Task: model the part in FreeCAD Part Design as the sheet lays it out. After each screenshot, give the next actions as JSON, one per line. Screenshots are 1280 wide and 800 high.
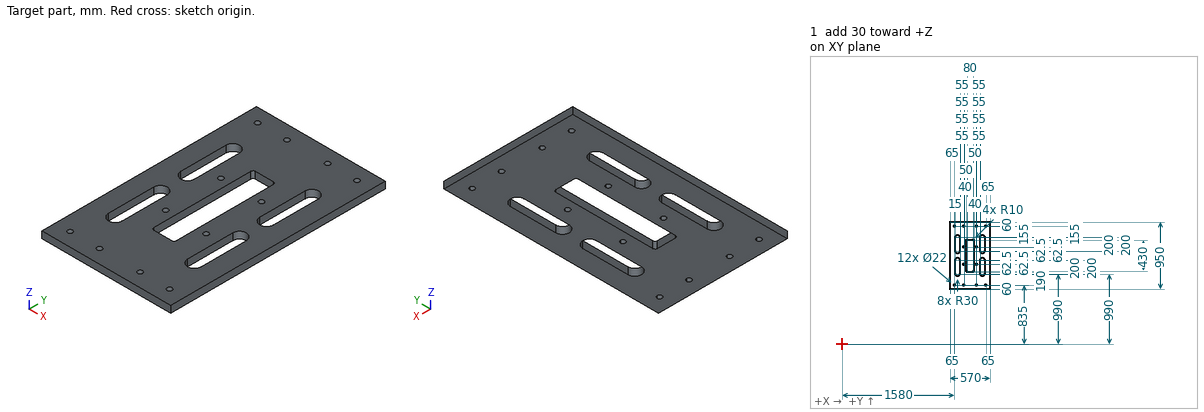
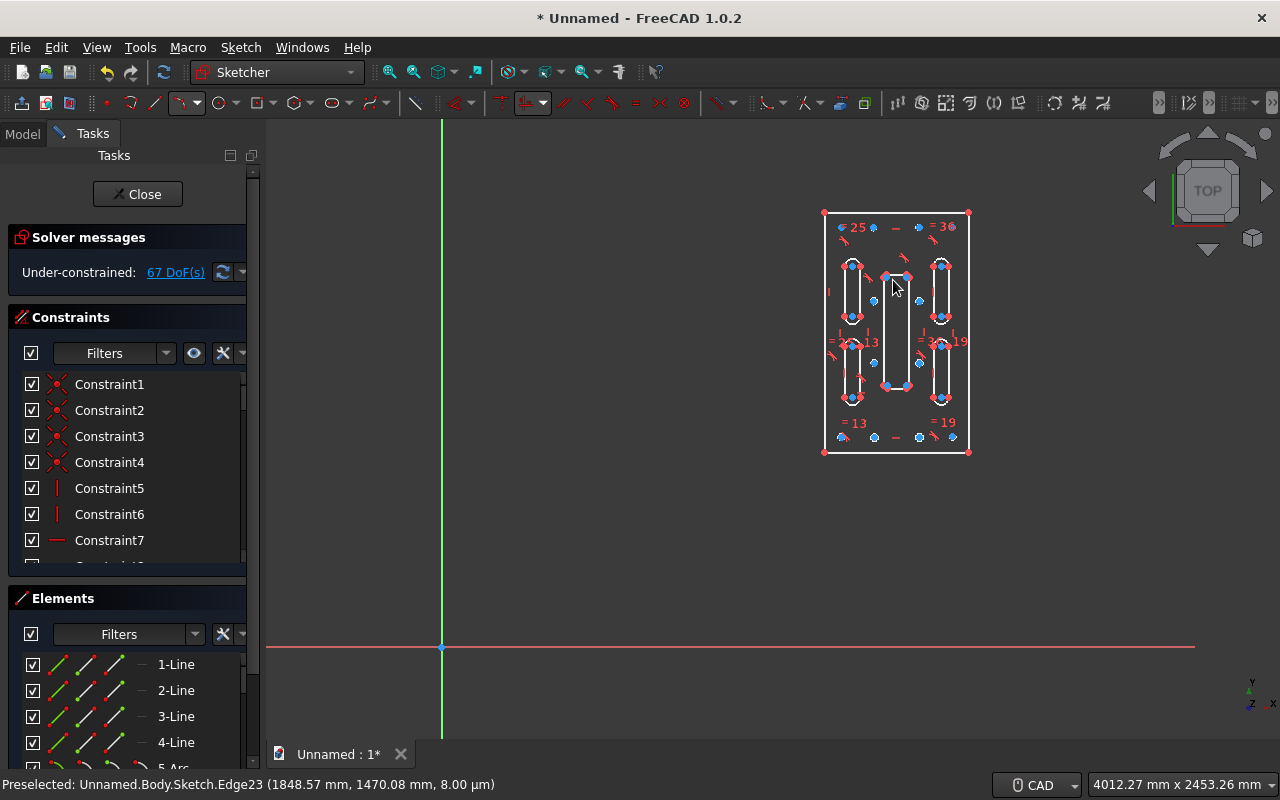
{"action": "scroll", "coordinate": [909, 310], "scroll_direction": "up", "scroll_amount": 2}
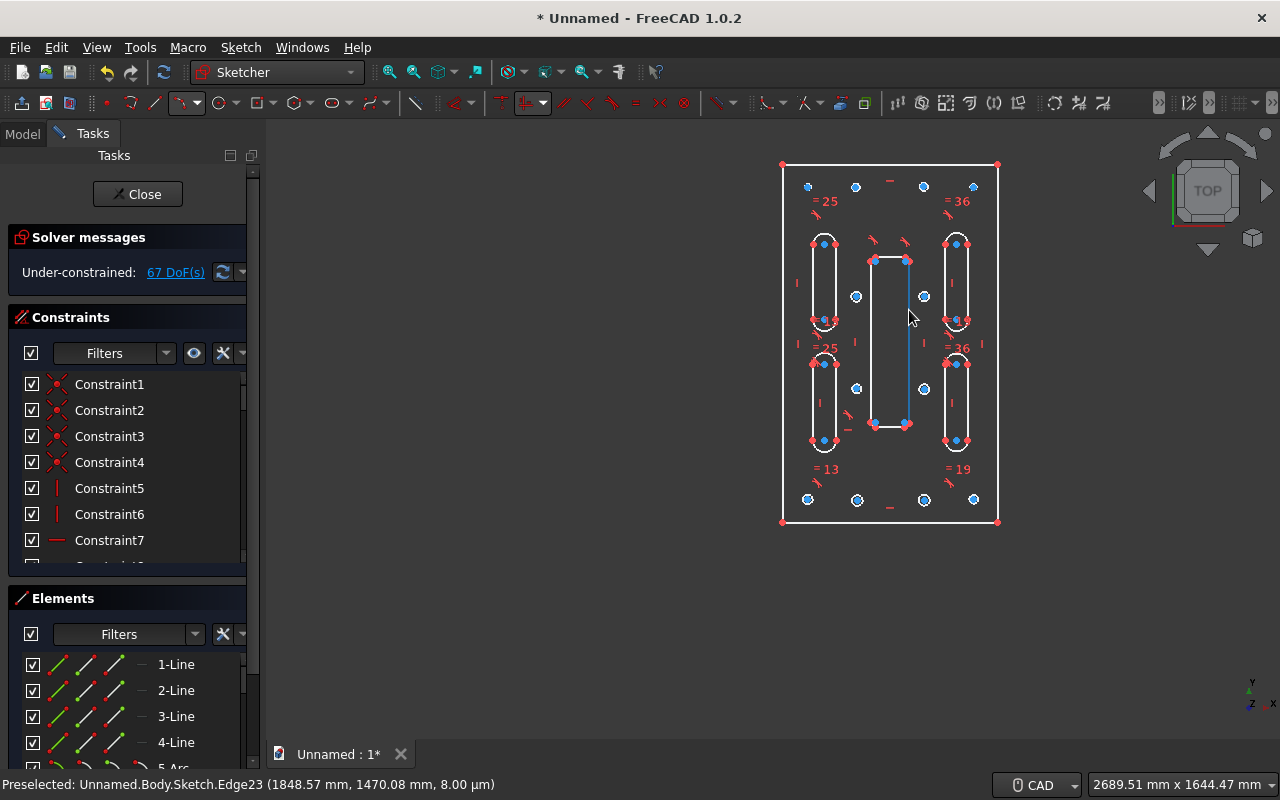
{"action": "left_click", "coordinate": [909, 310]}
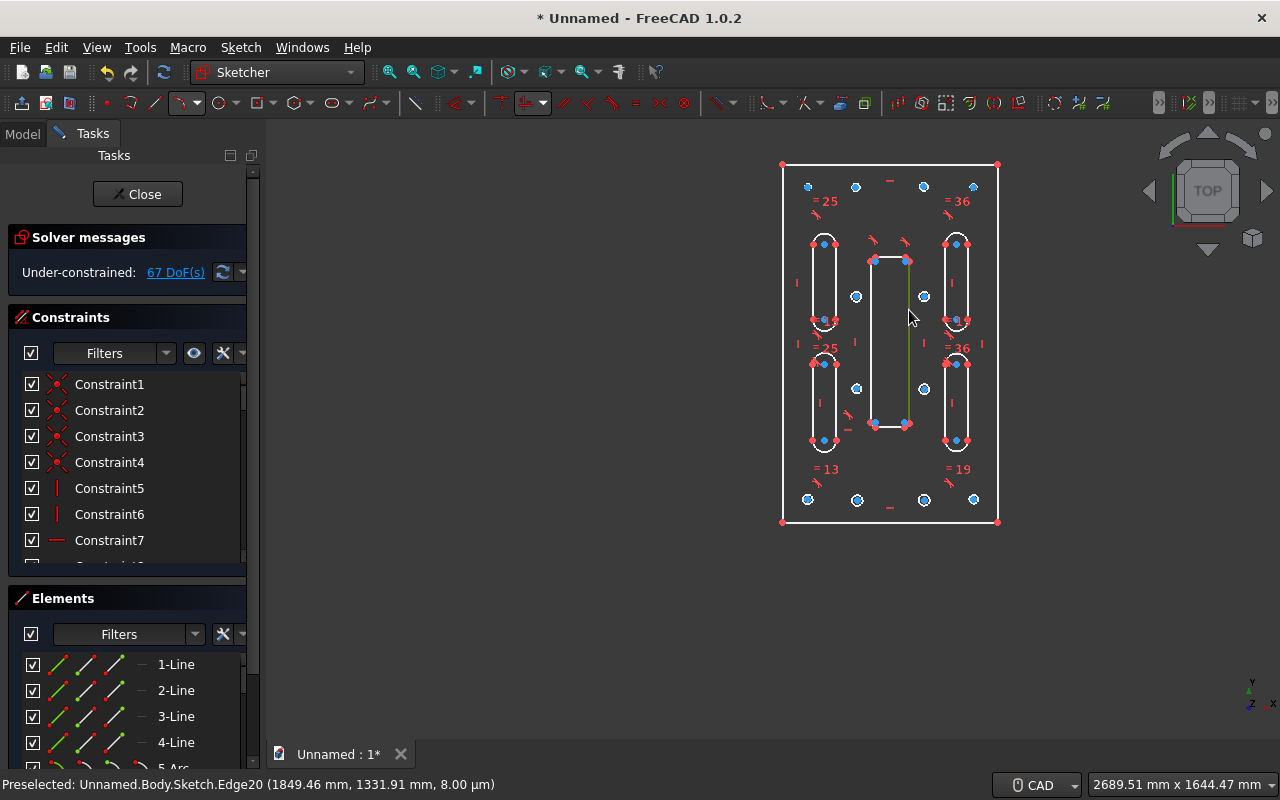
{"action": "scroll", "coordinate": [908, 258], "scroll_direction": "up", "scroll_amount": 8}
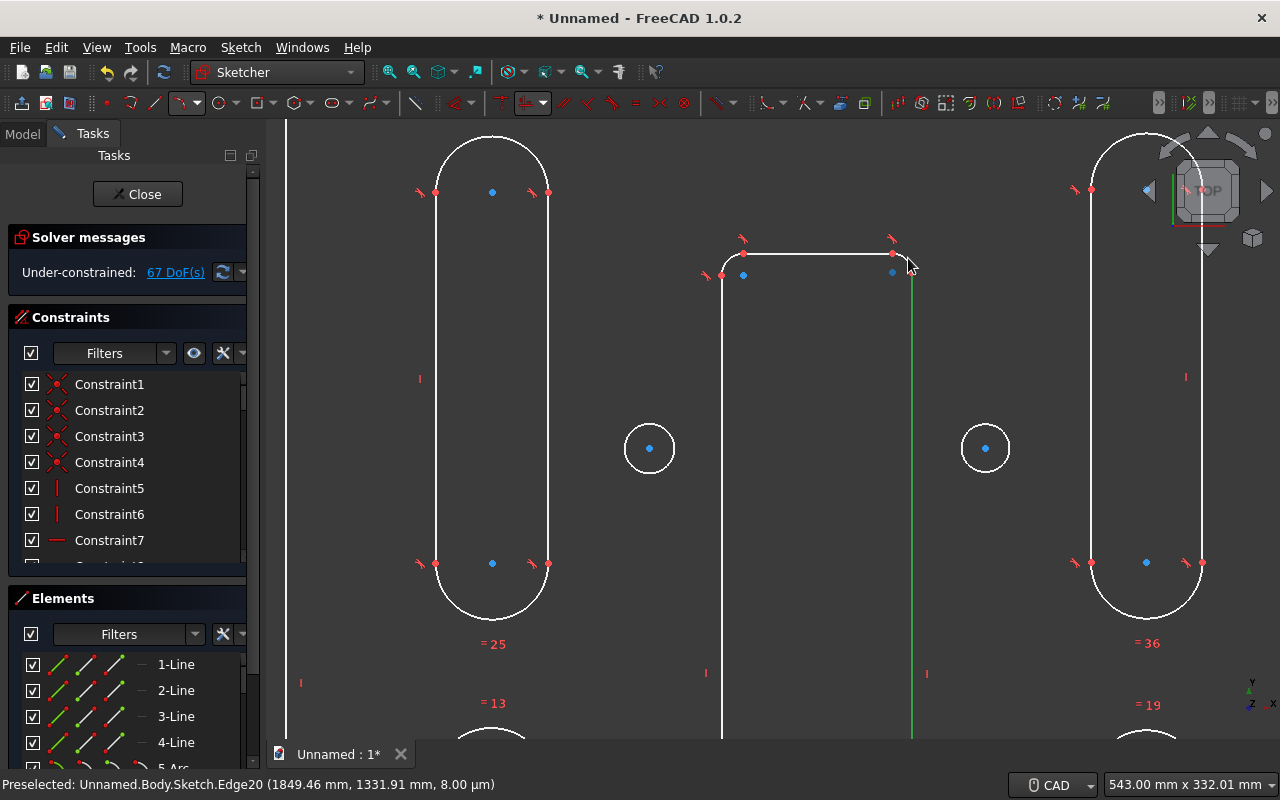
{"action": "left_click", "coordinate": [906, 259]}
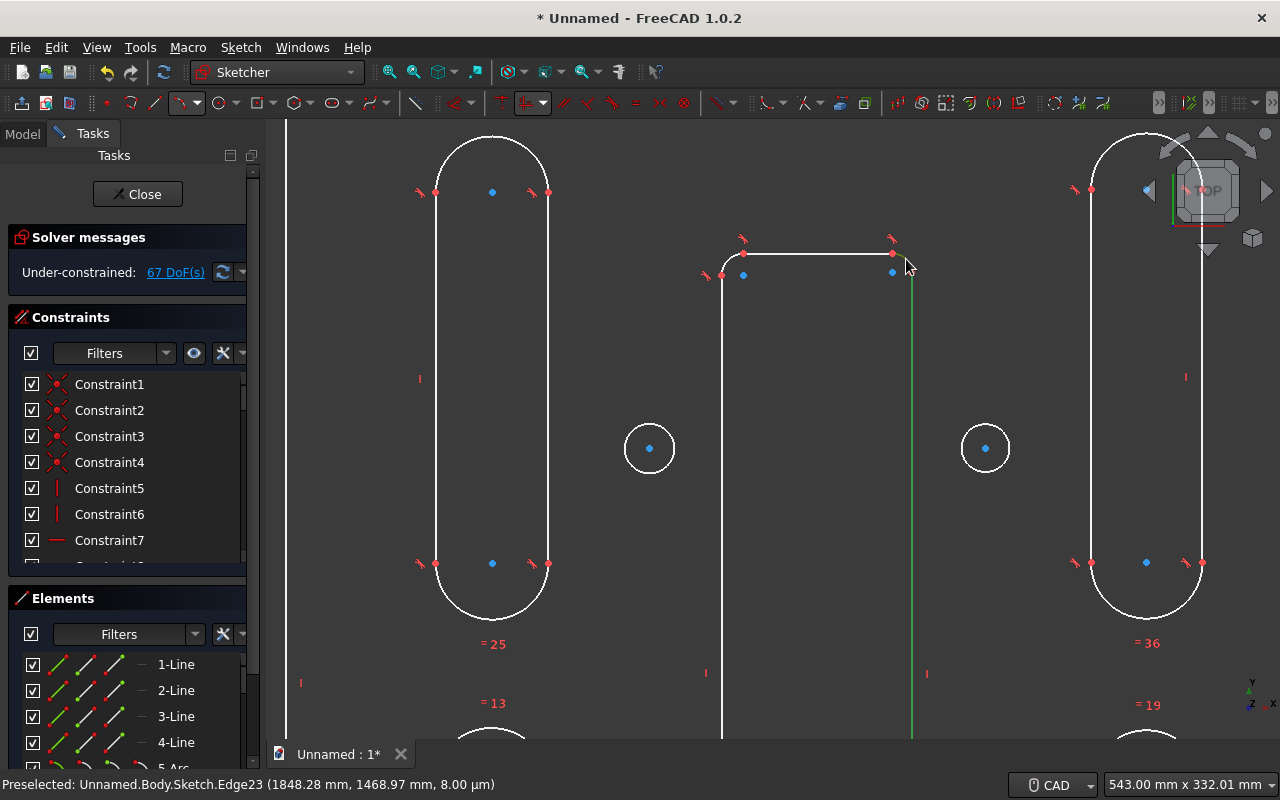
{"action": "left_click", "coordinate": [612, 104]}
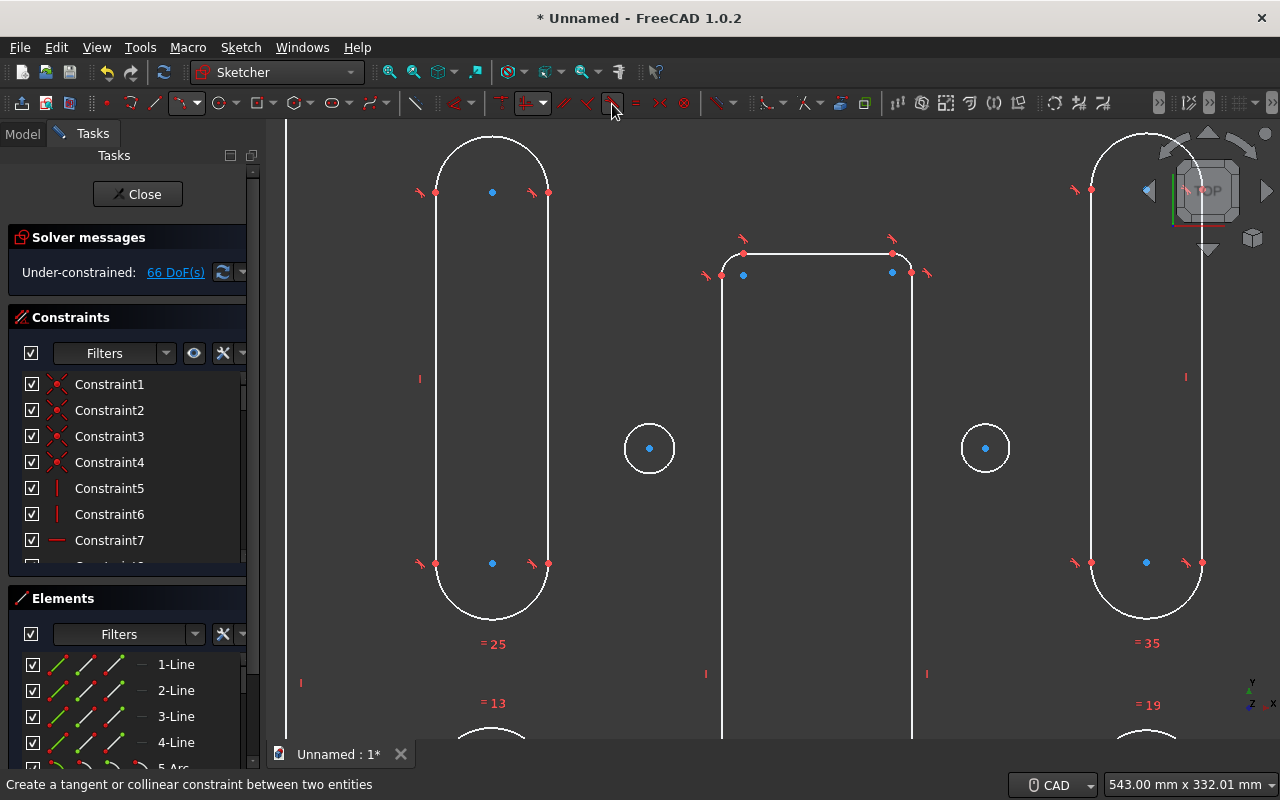
{"action": "scroll", "coordinate": [908, 278], "scroll_direction": "down", "scroll_amount": 10}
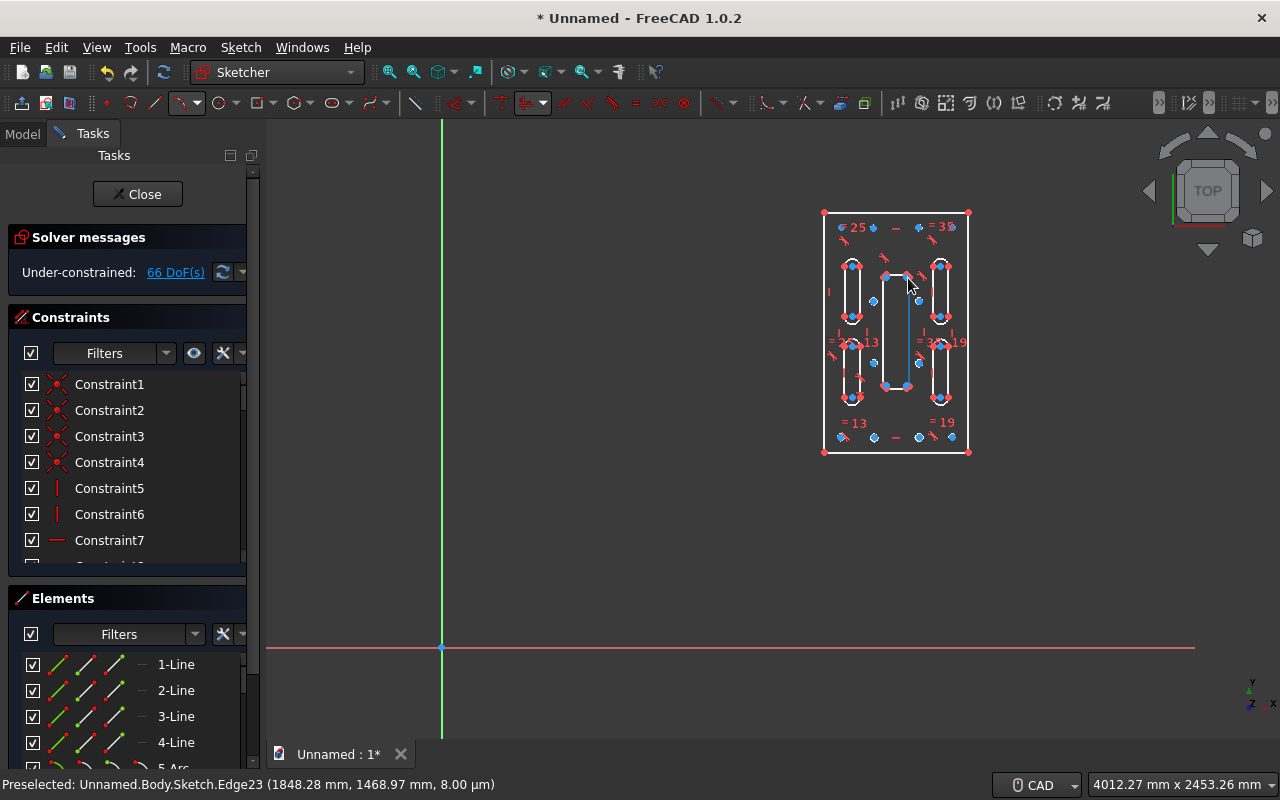
{"action": "scroll", "coordinate": [909, 310], "scroll_direction": "up", "scroll_amount": 2}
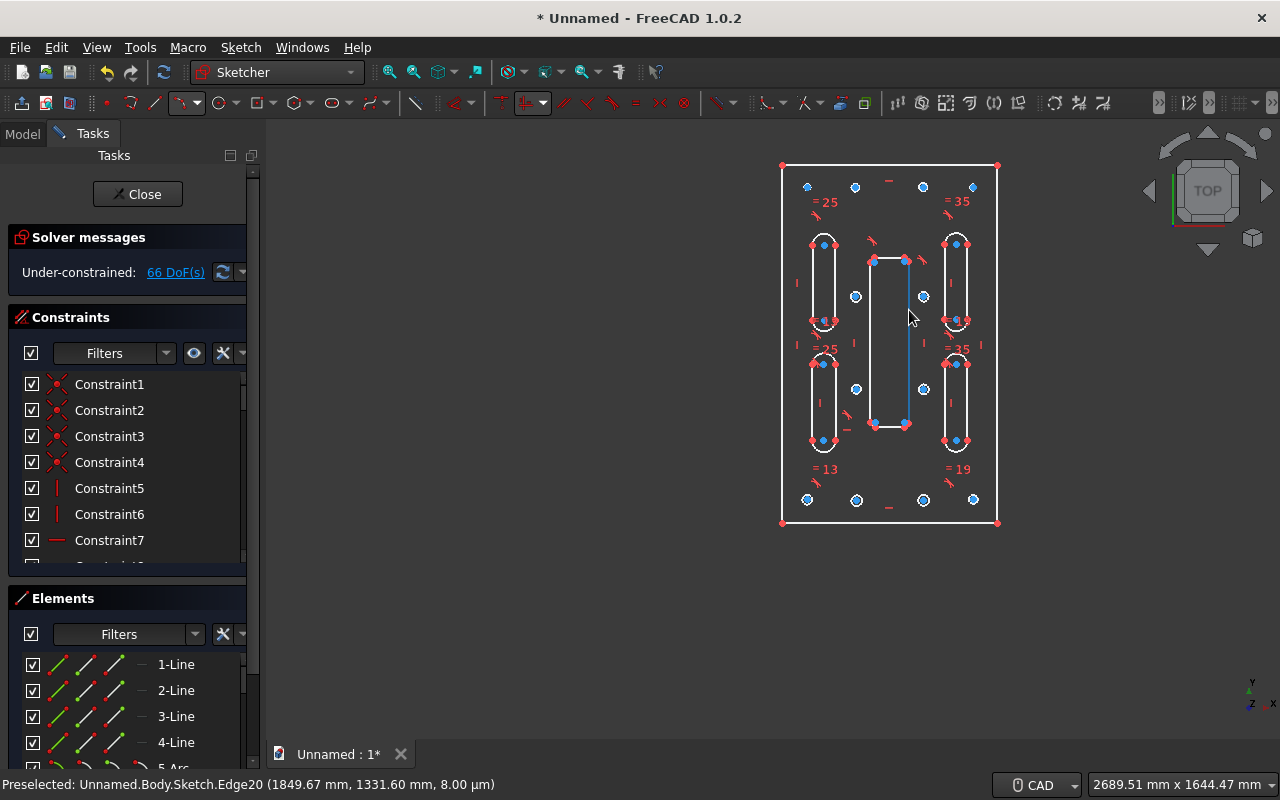
{"action": "left_click", "coordinate": [909, 310]}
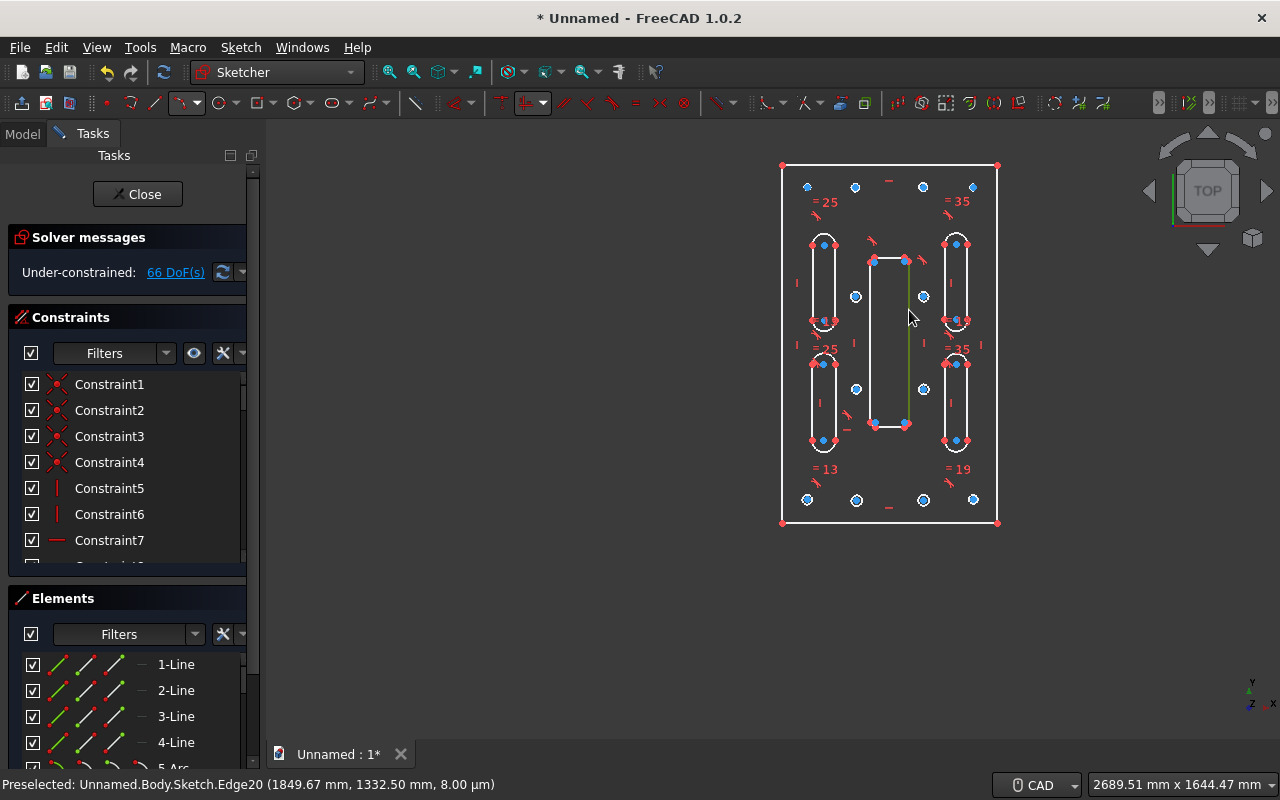
{"action": "scroll", "coordinate": [907, 426], "scroll_direction": "up", "scroll_amount": 8}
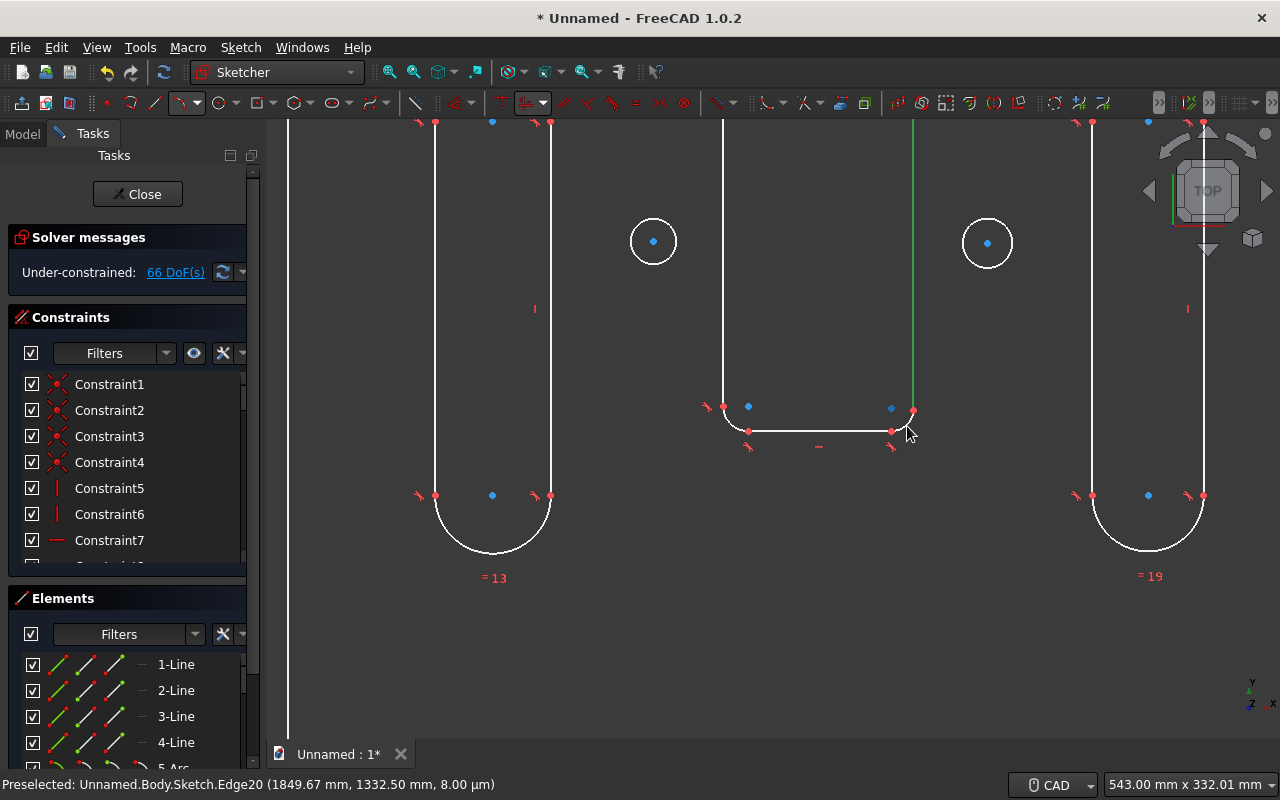
{"action": "left_click", "coordinate": [906, 425]}